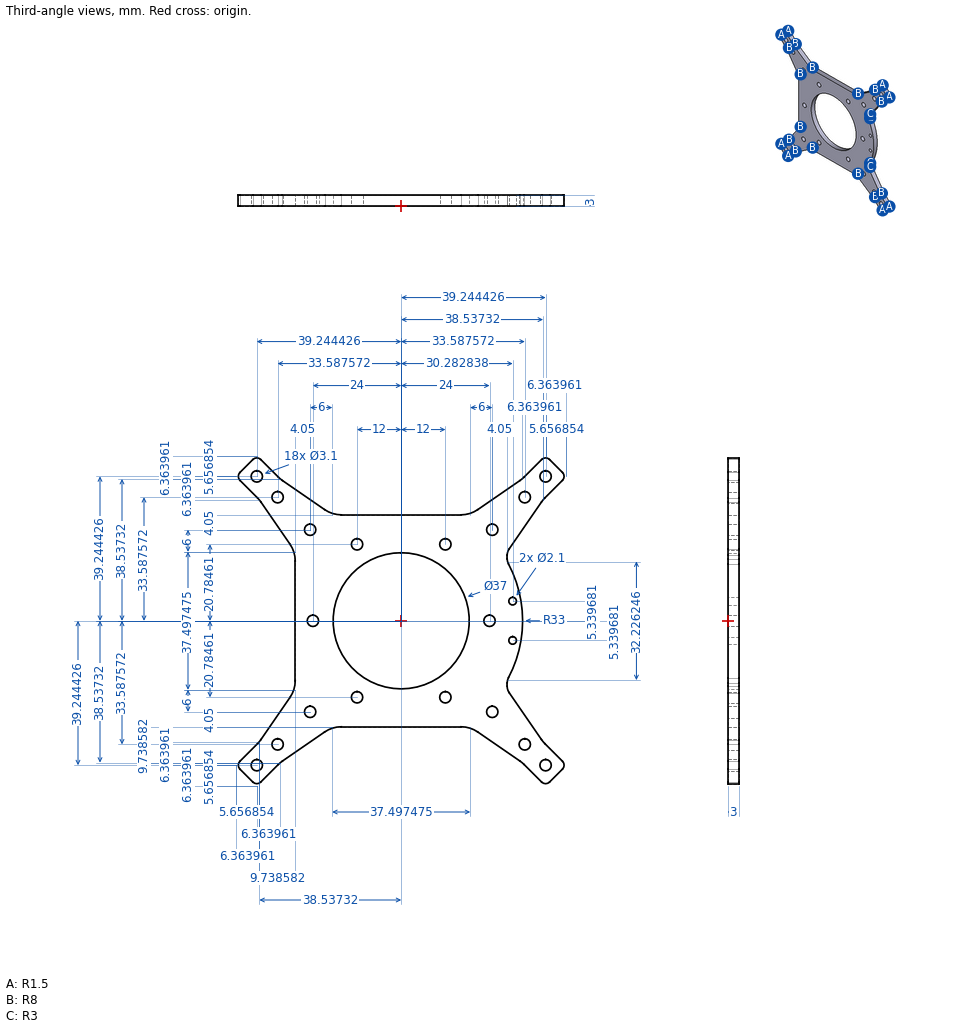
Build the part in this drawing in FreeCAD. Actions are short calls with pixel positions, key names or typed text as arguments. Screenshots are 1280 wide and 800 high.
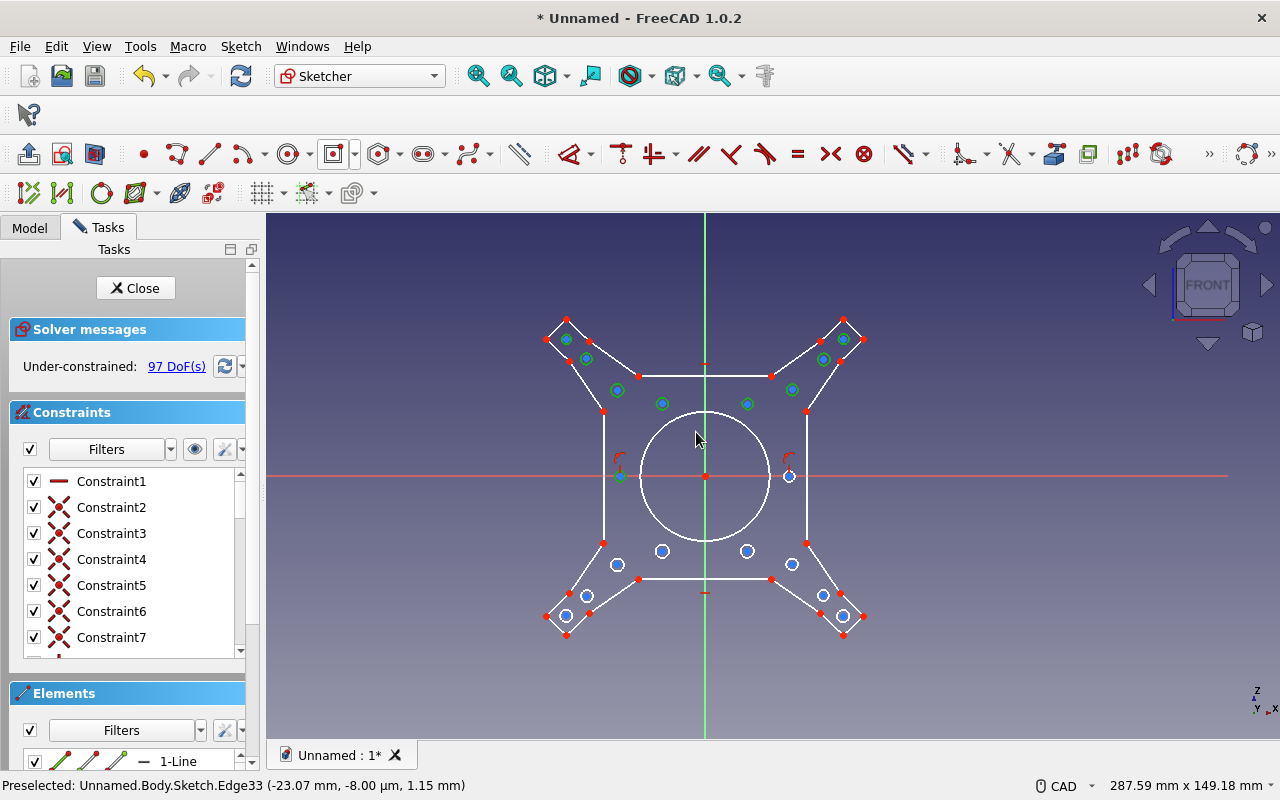
scroll(622, 560, up, 4)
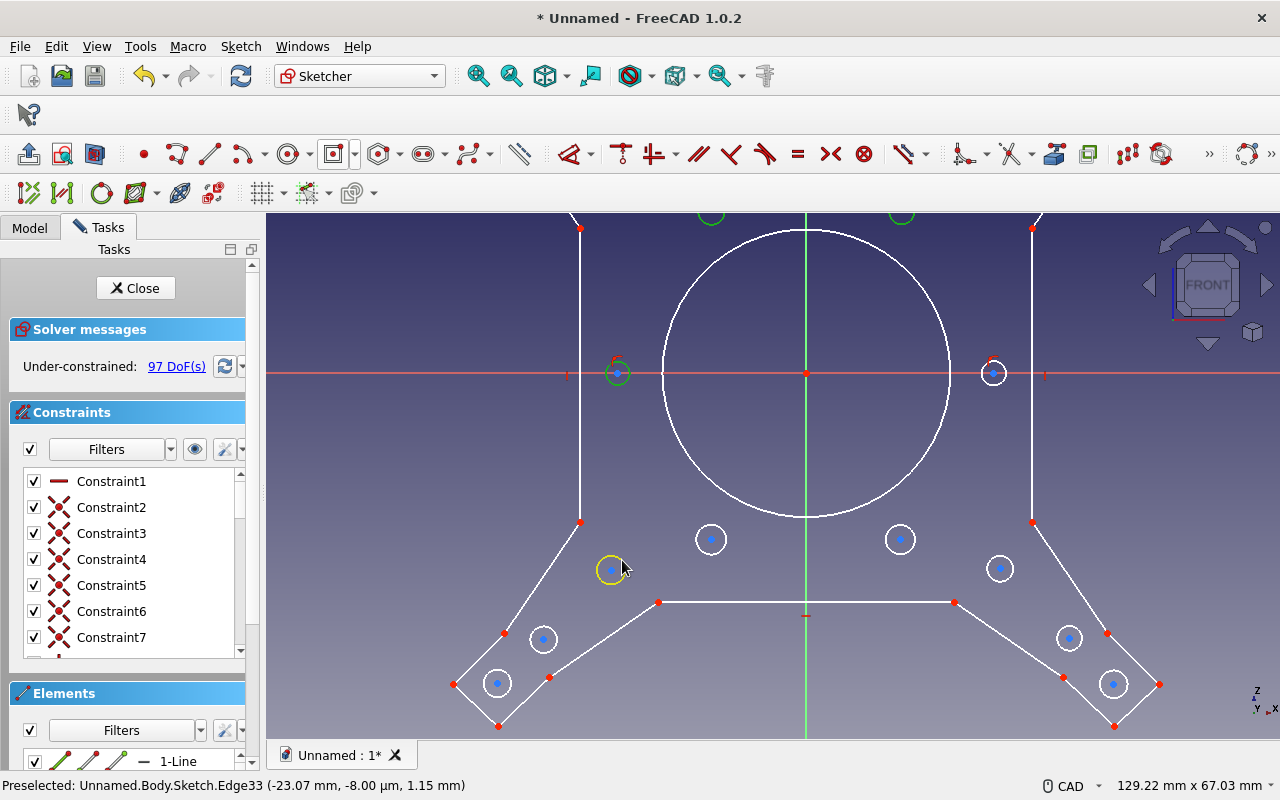
click(621, 560)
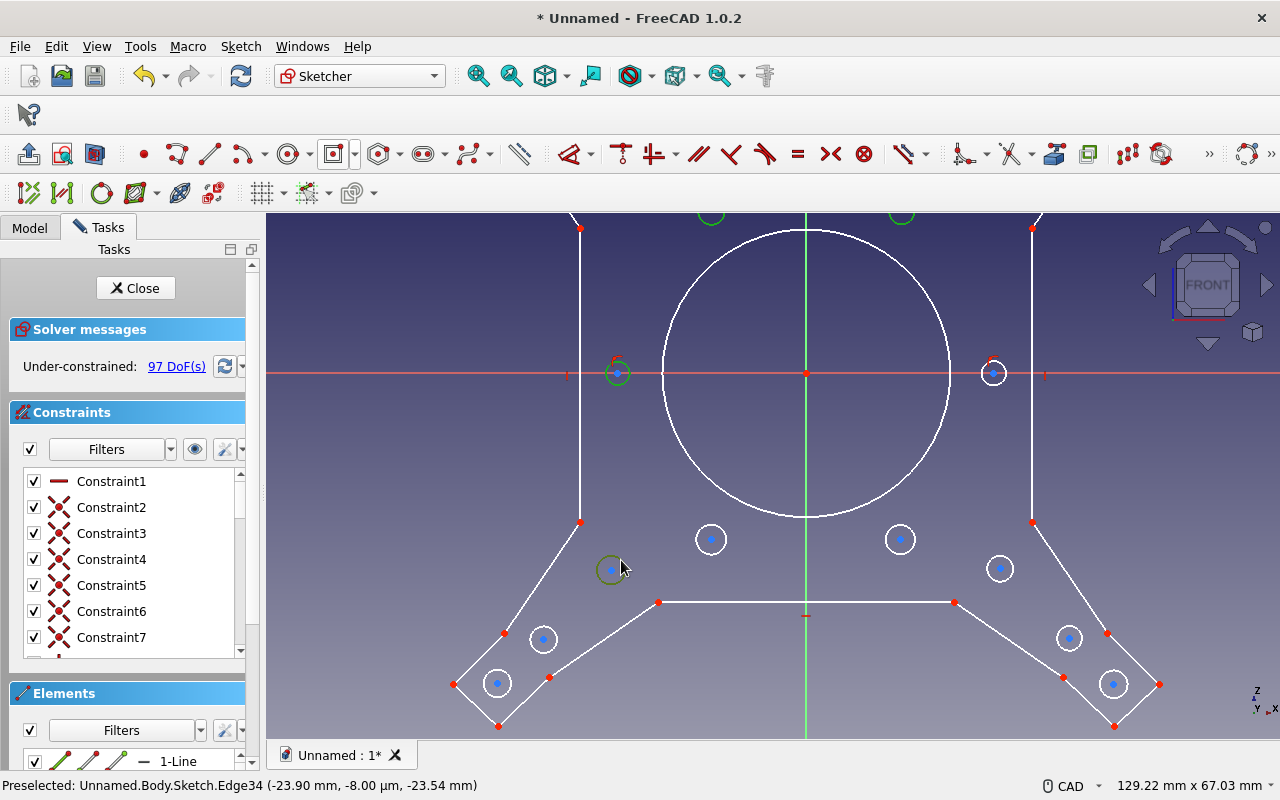
click(553, 630)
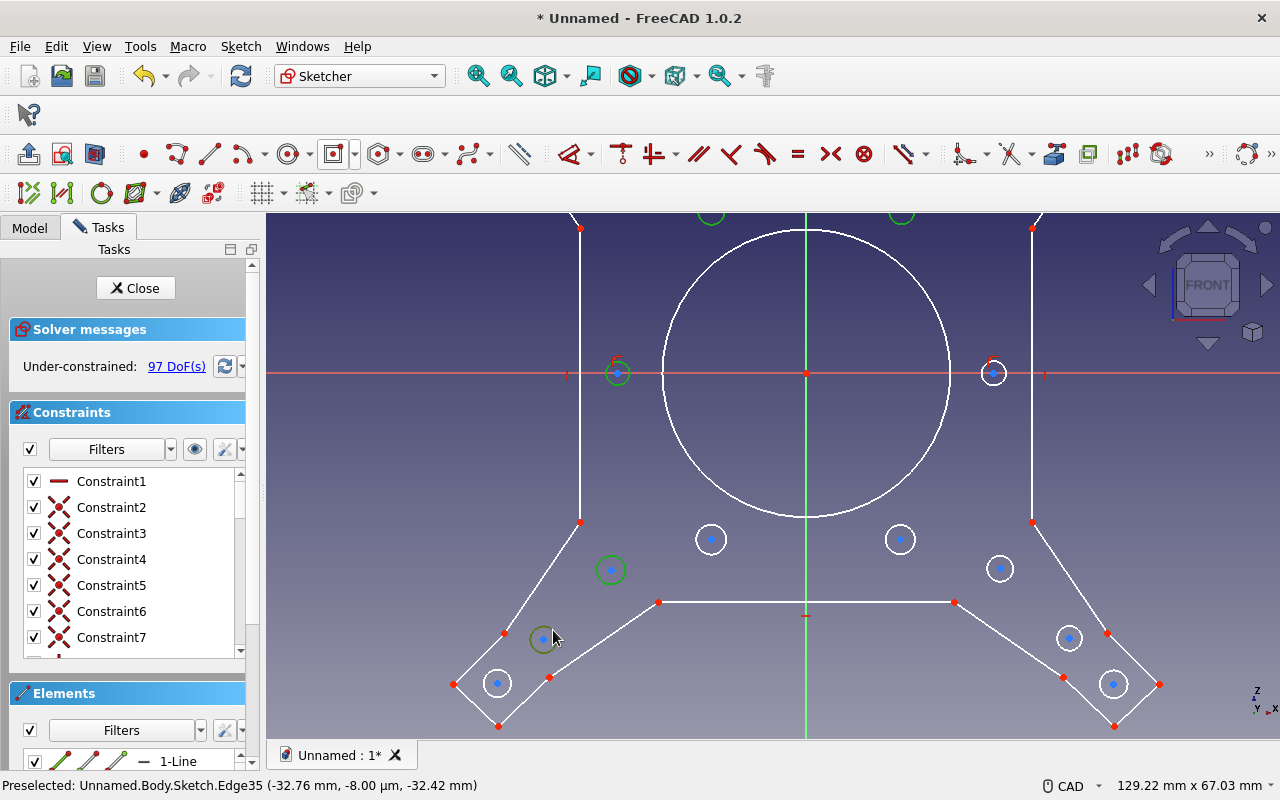
click(507, 674)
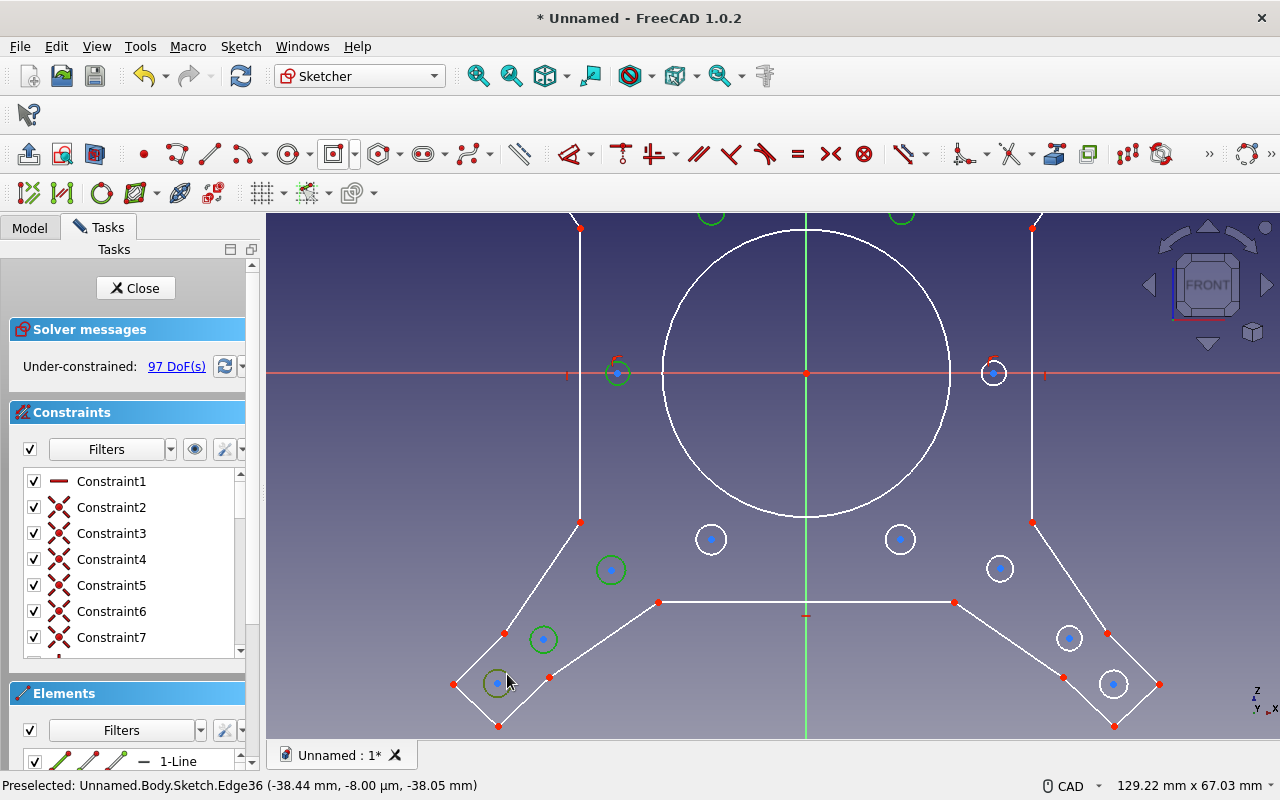
click(722, 529)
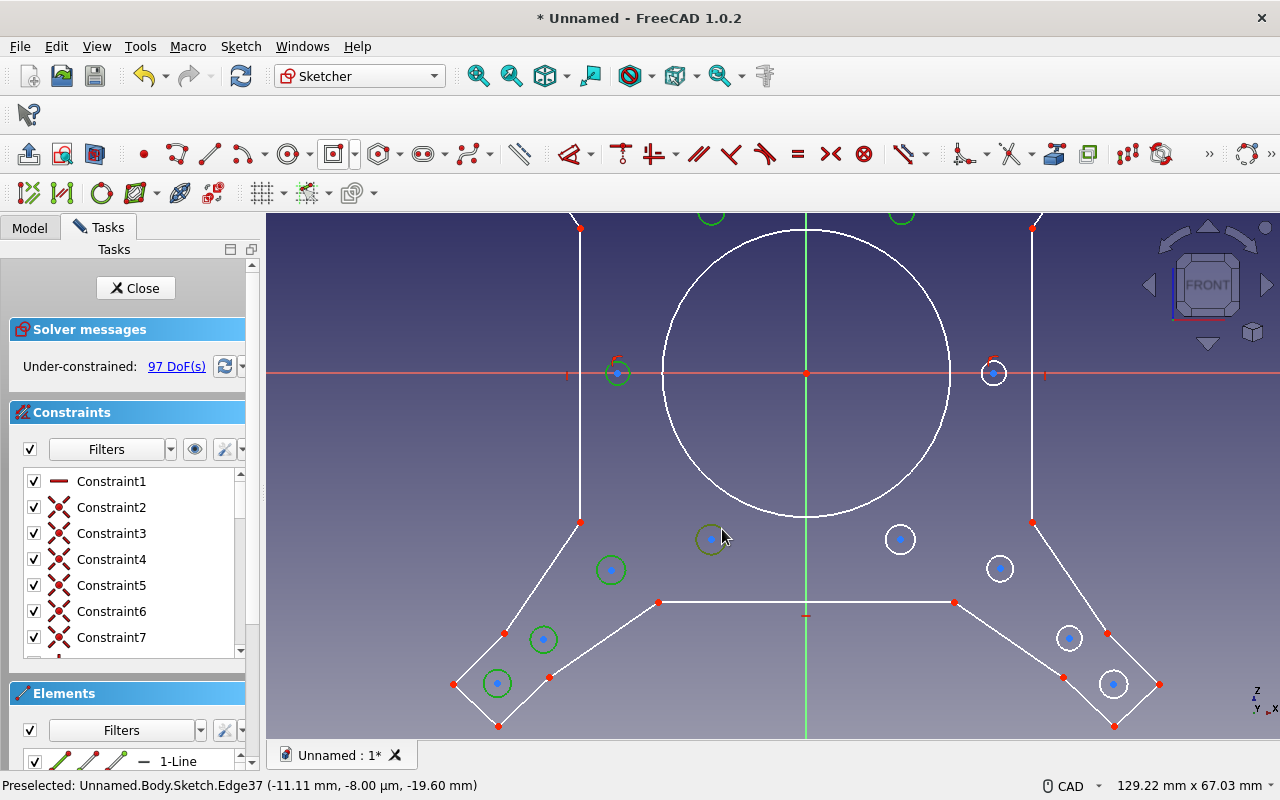
click(982, 373)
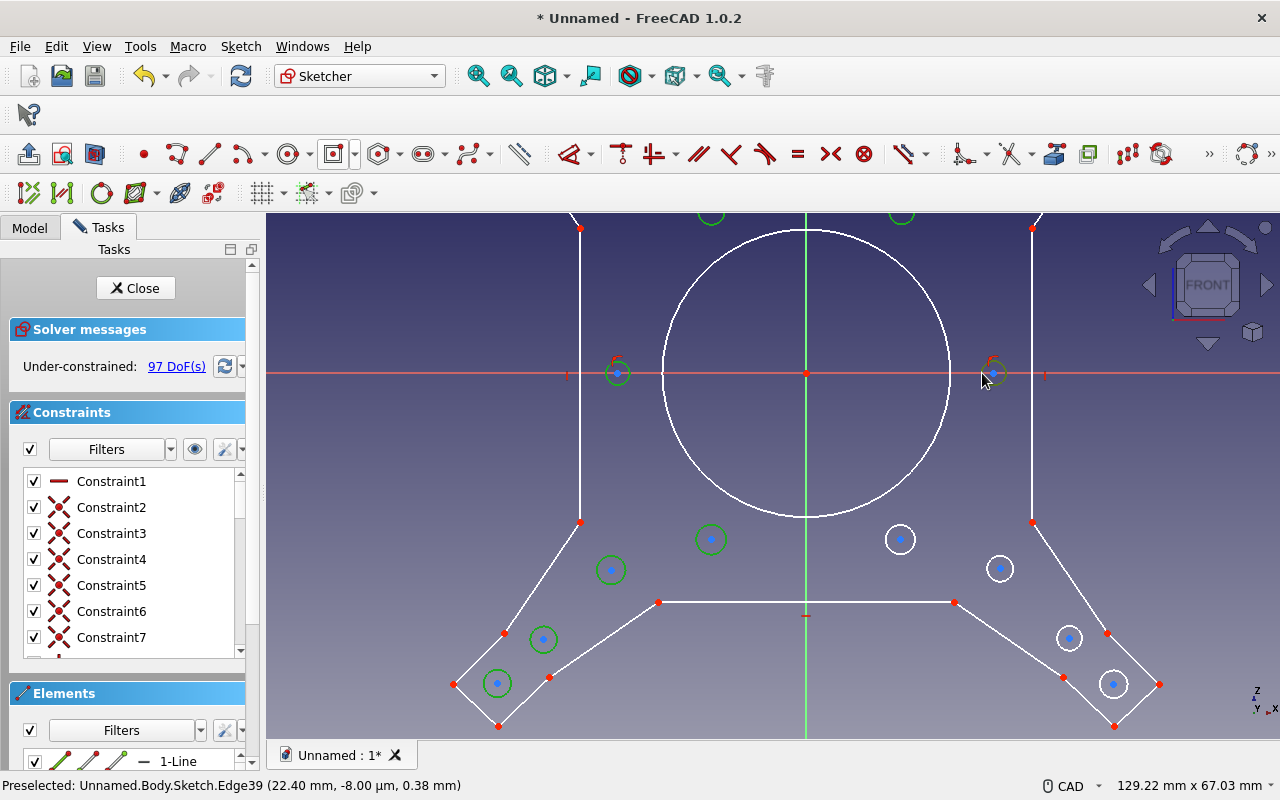
click(911, 529)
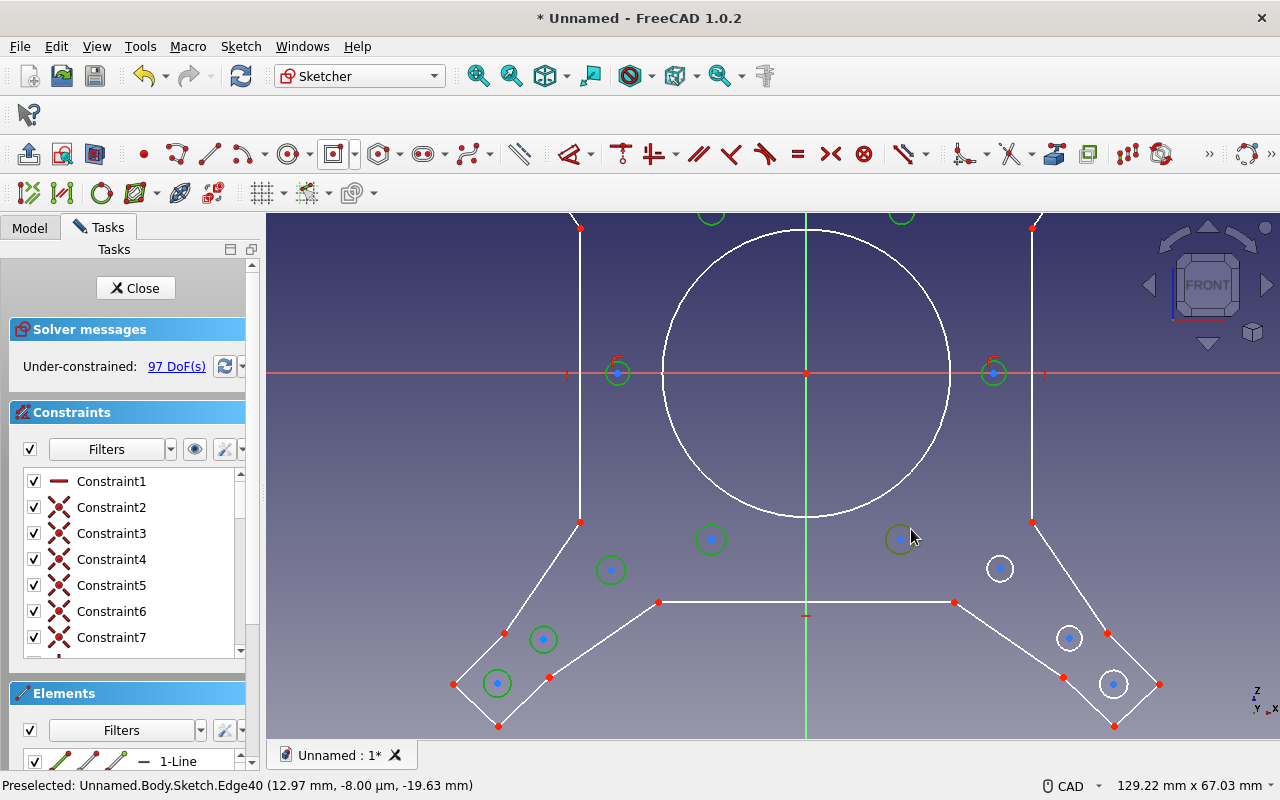
click(1009, 560)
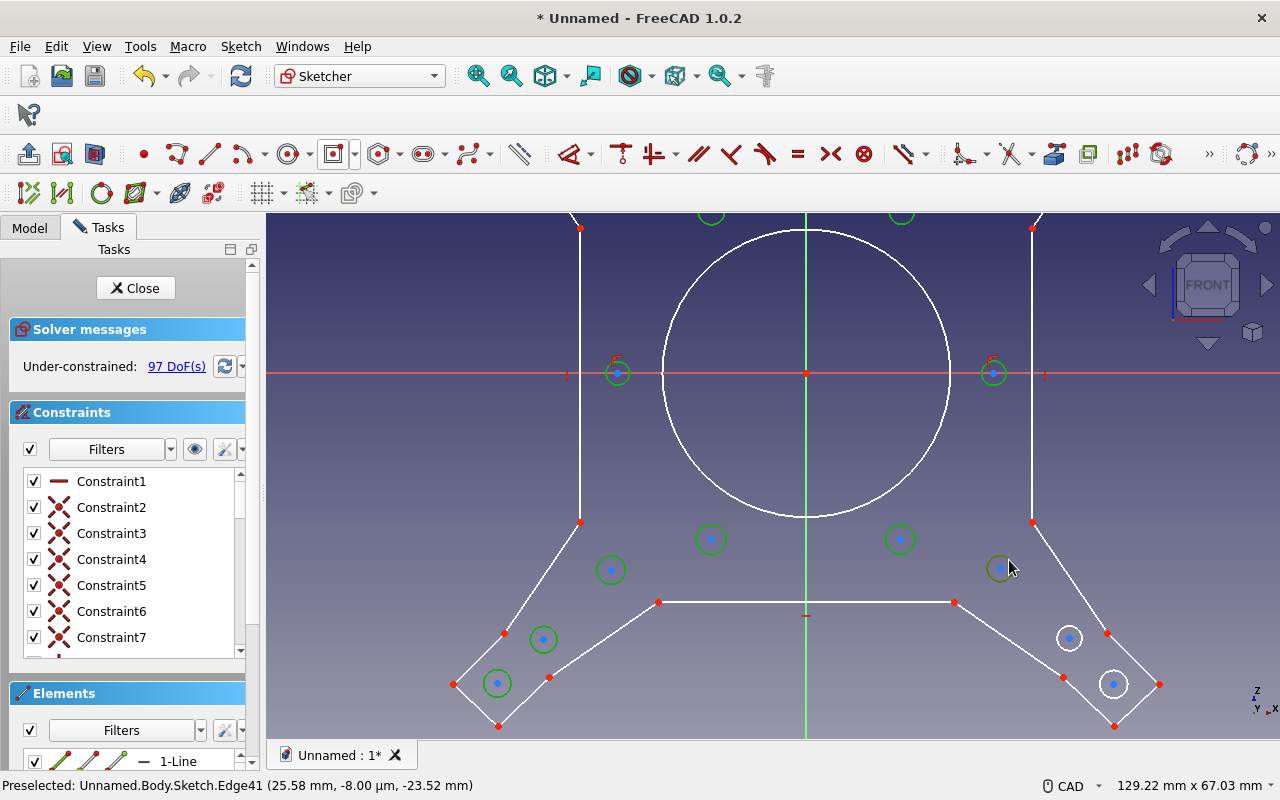
click(1078, 630)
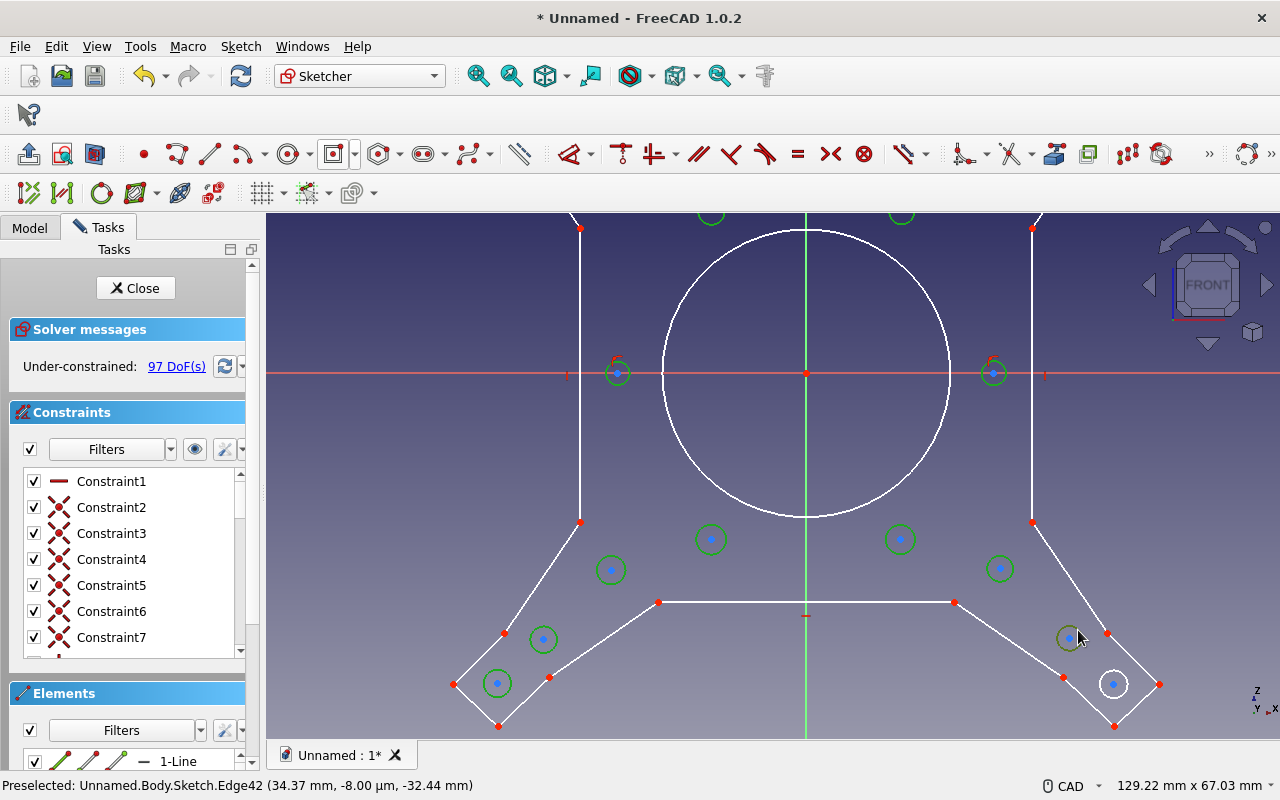
click(1104, 675)